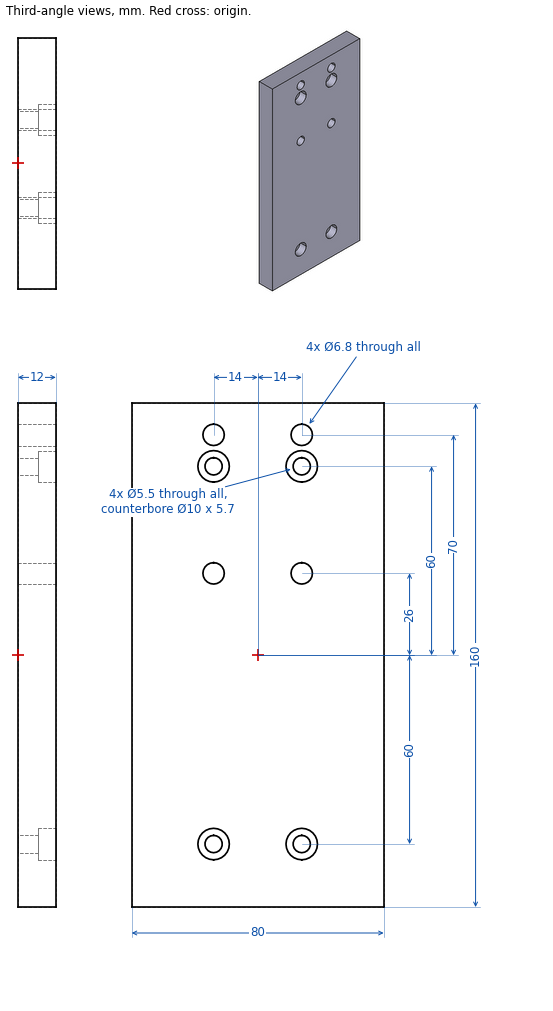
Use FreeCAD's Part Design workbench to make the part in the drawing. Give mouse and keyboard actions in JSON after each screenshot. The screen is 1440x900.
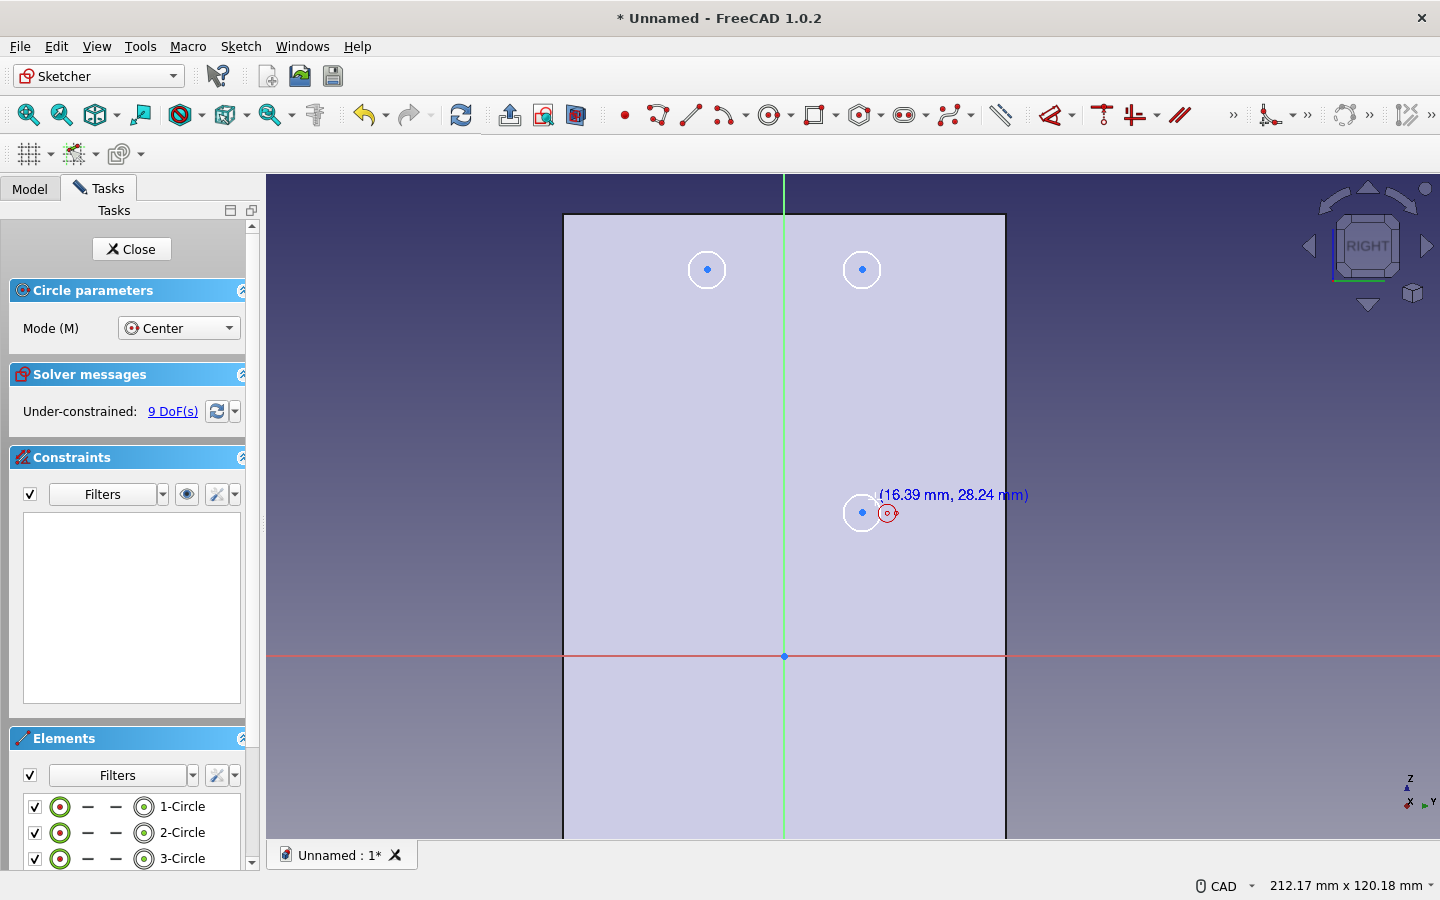
{"action": "left_click", "coordinate": [707, 512]}
{"action": "left_click", "coordinate": [720, 499]}
{"action": "key", "text": "Escape"}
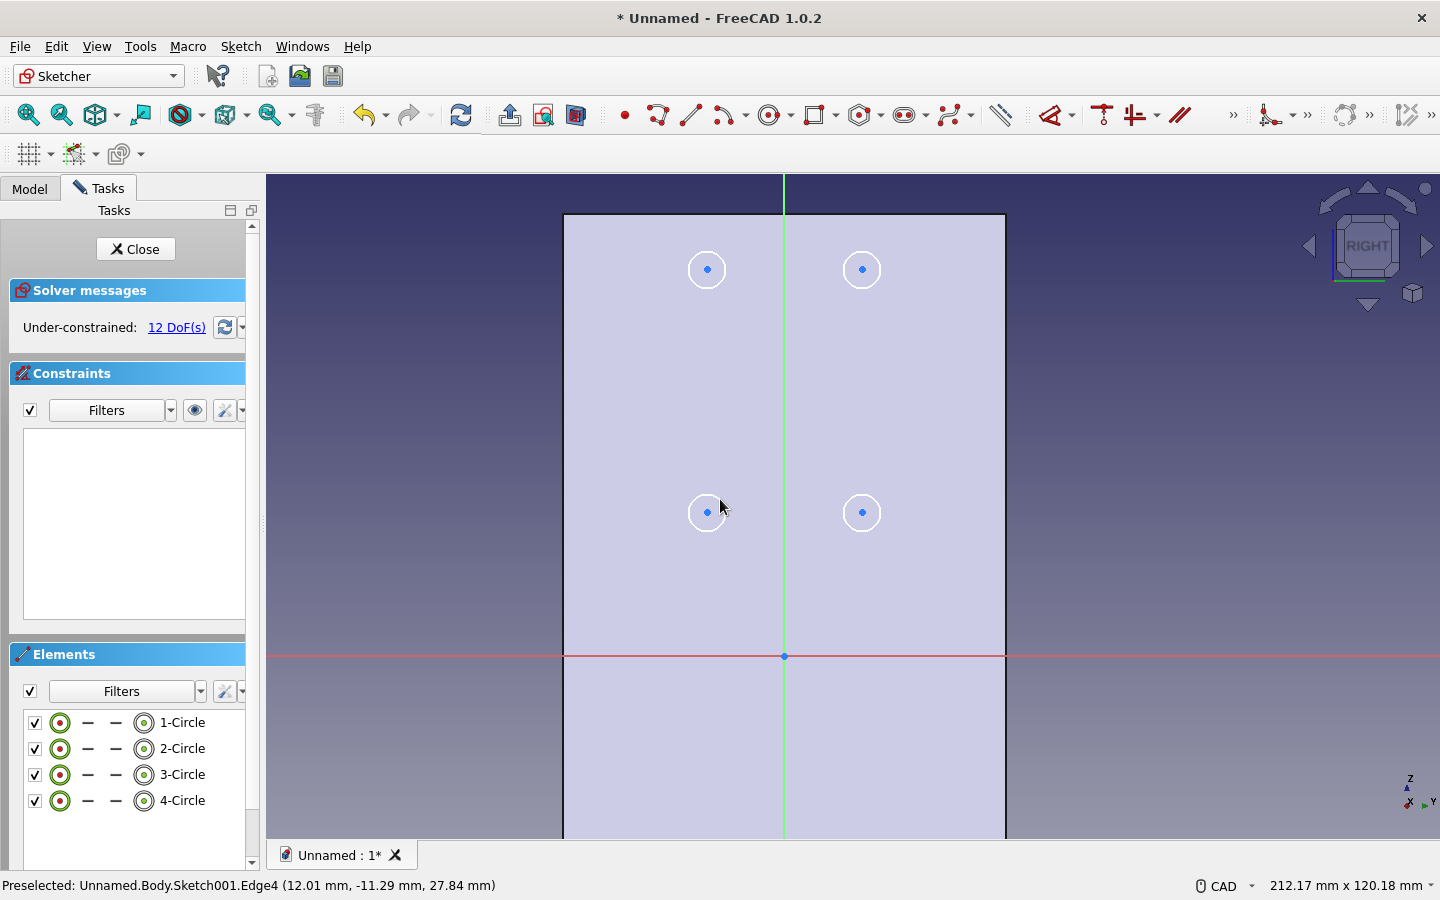
{"action": "left_click", "coordinate": [875, 257]}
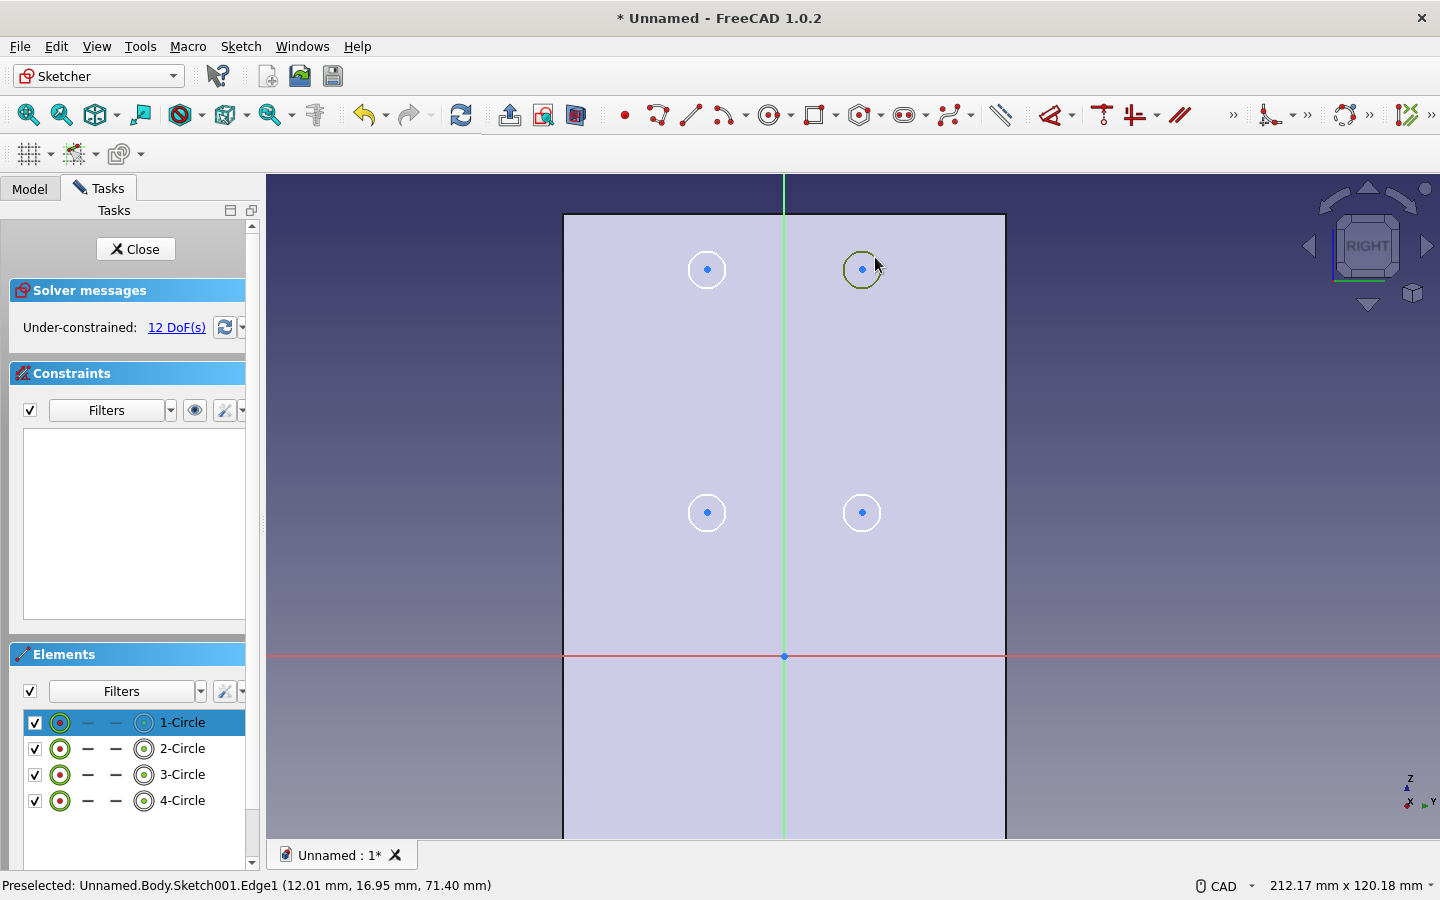
{"action": "left_click", "coordinate": [720, 257]}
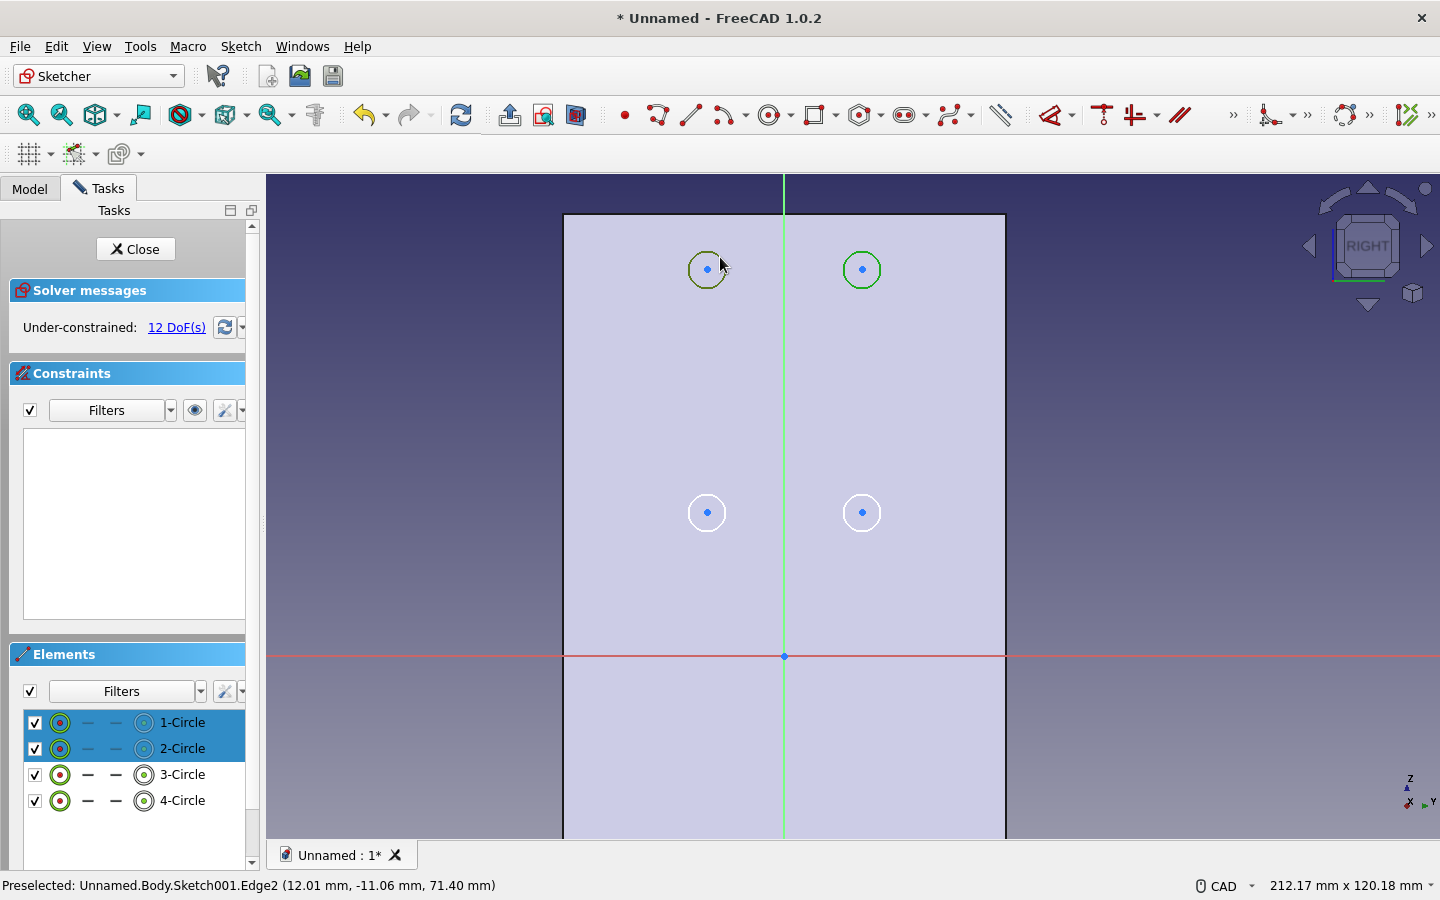
{"action": "left_click", "coordinate": [875, 500]}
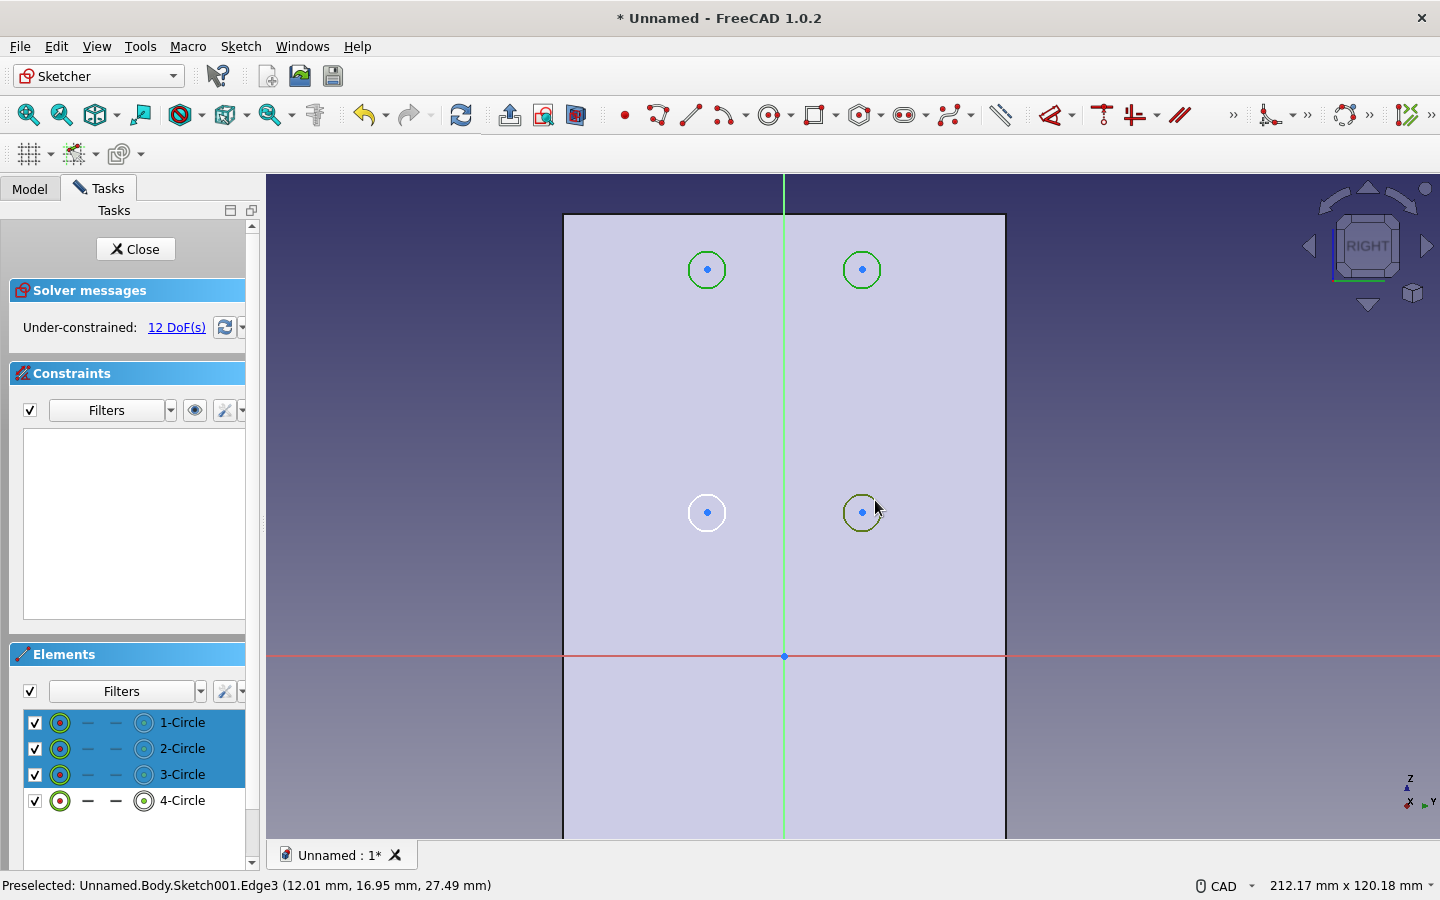
{"action": "left_click", "coordinate": [720, 500]}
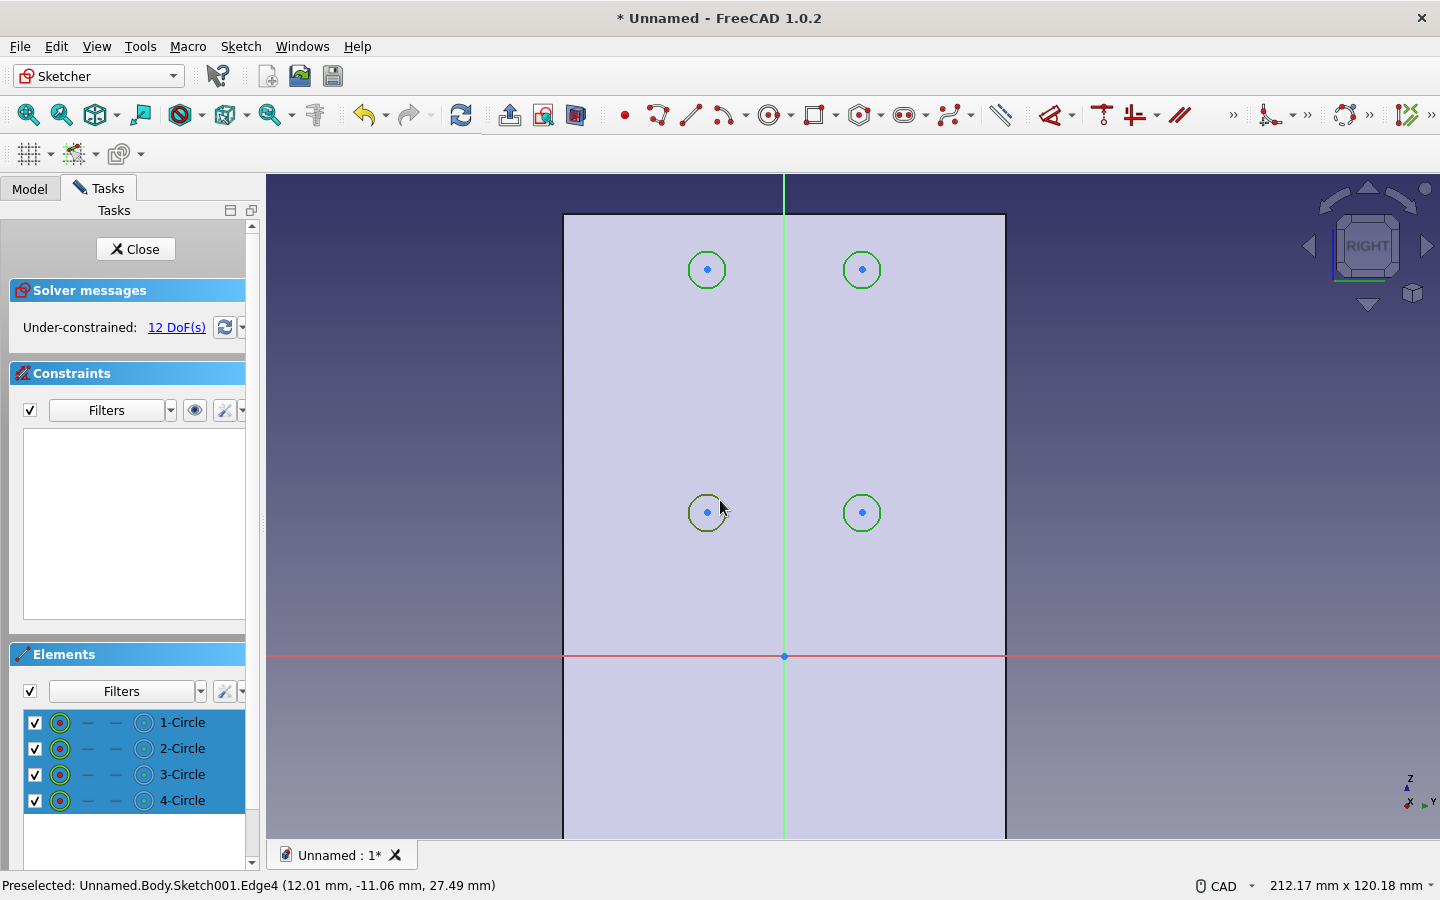
{"action": "key", "text": "e"}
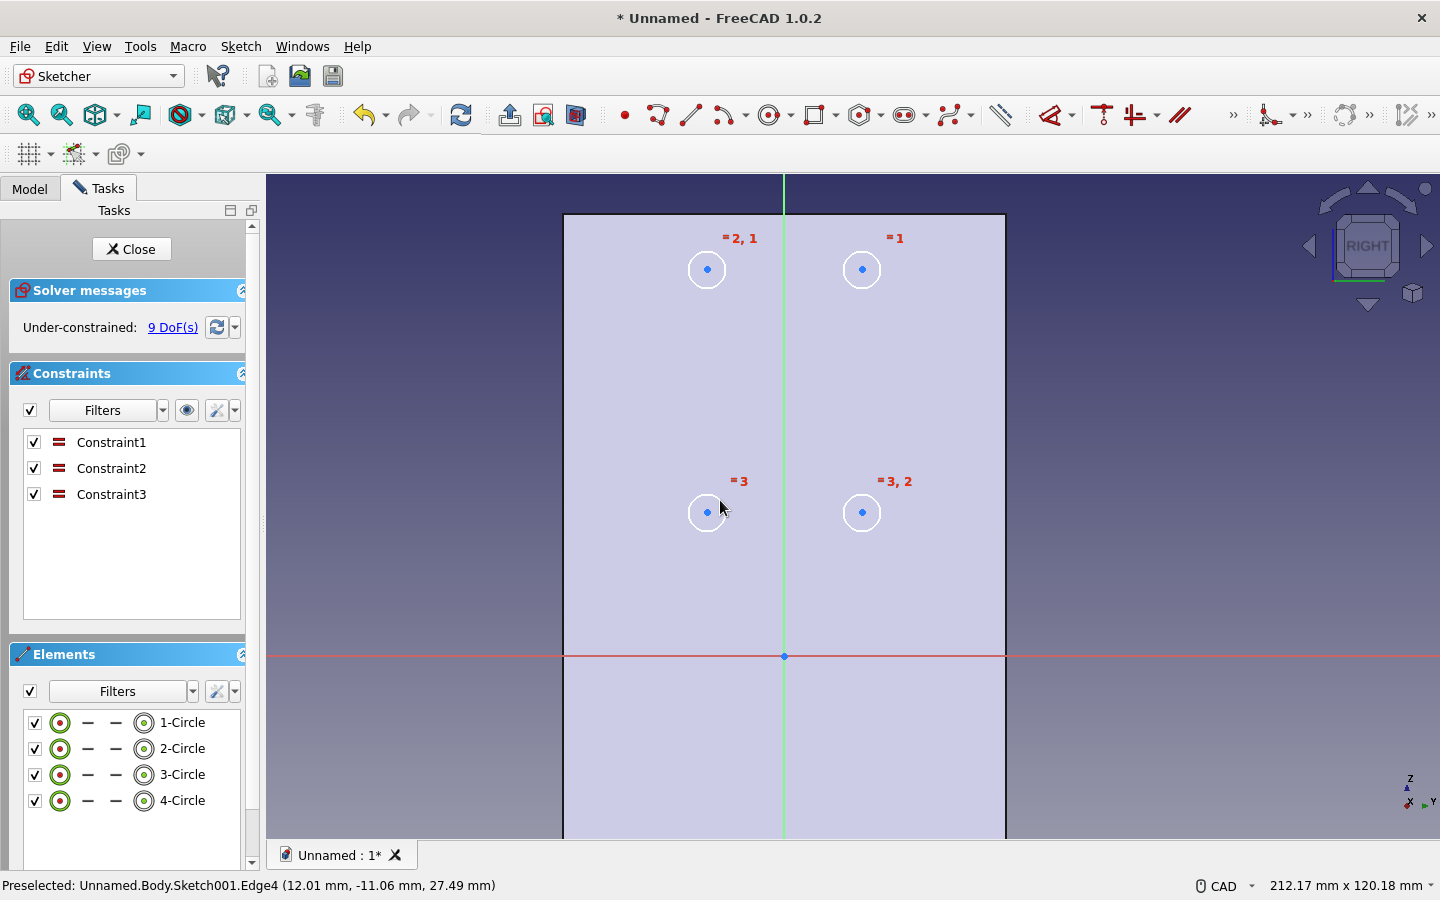
{"action": "left_click", "coordinate": [862, 270]}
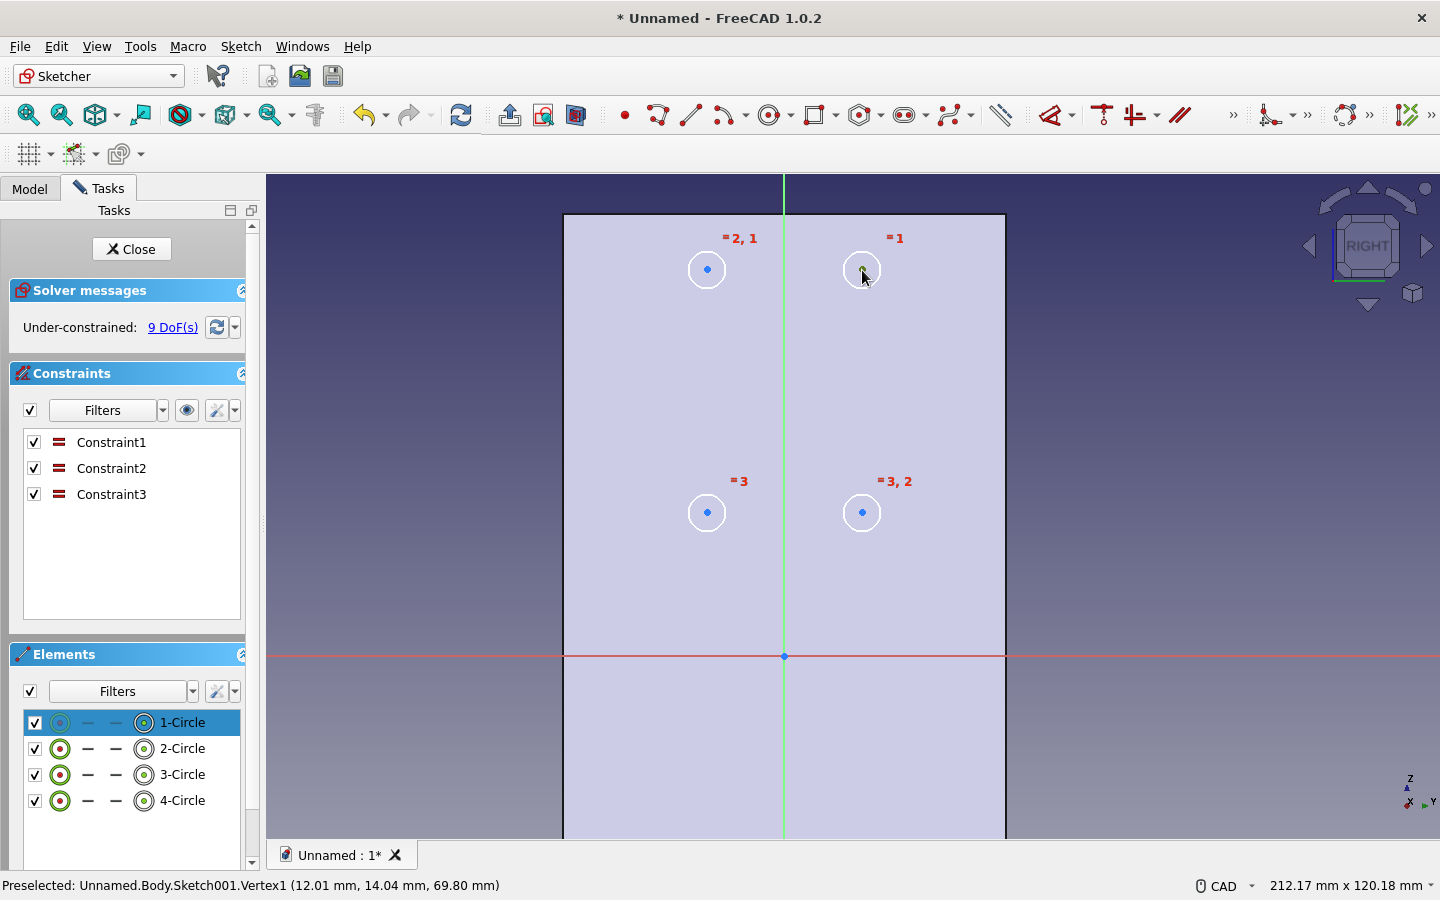
{"action": "left_click", "coordinate": [707, 270]}